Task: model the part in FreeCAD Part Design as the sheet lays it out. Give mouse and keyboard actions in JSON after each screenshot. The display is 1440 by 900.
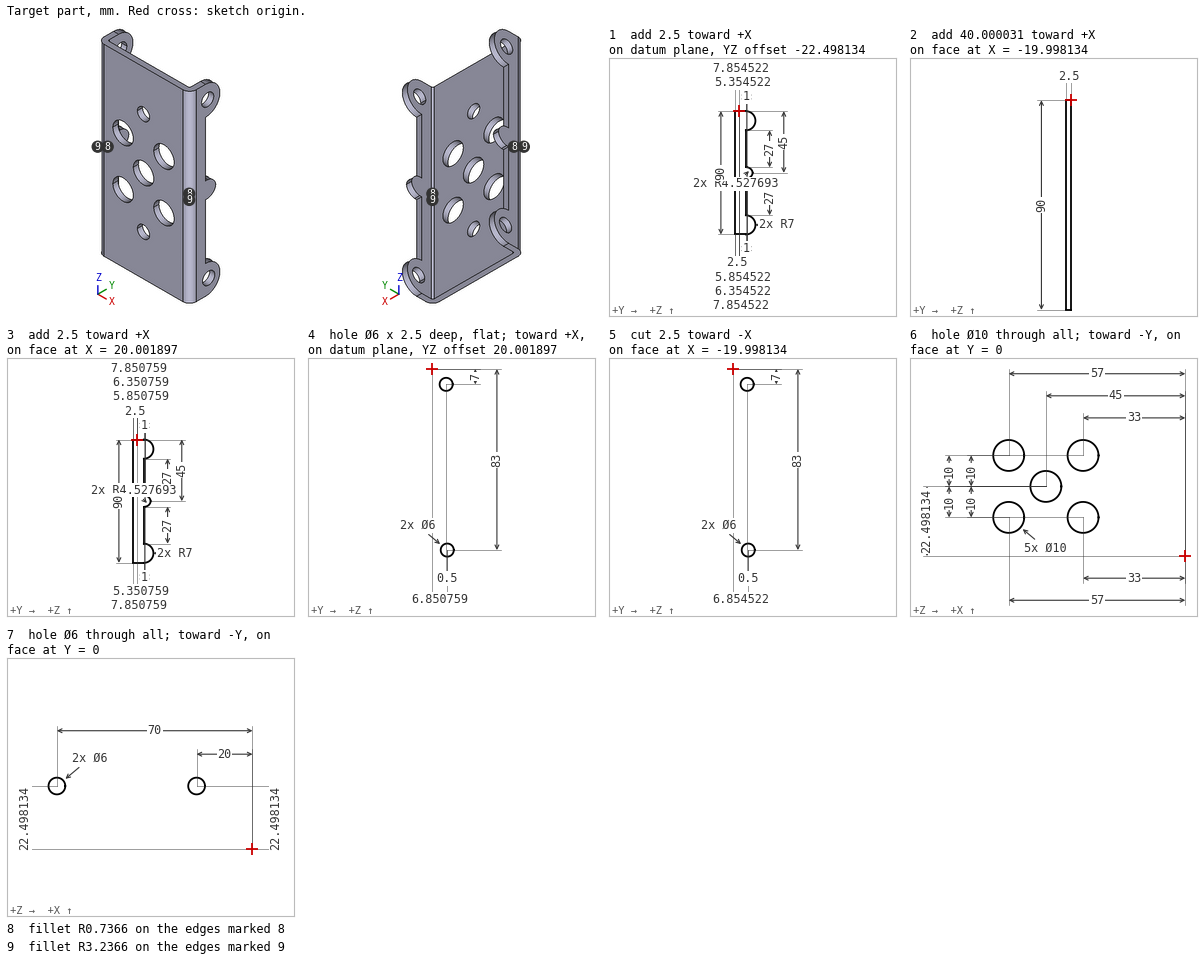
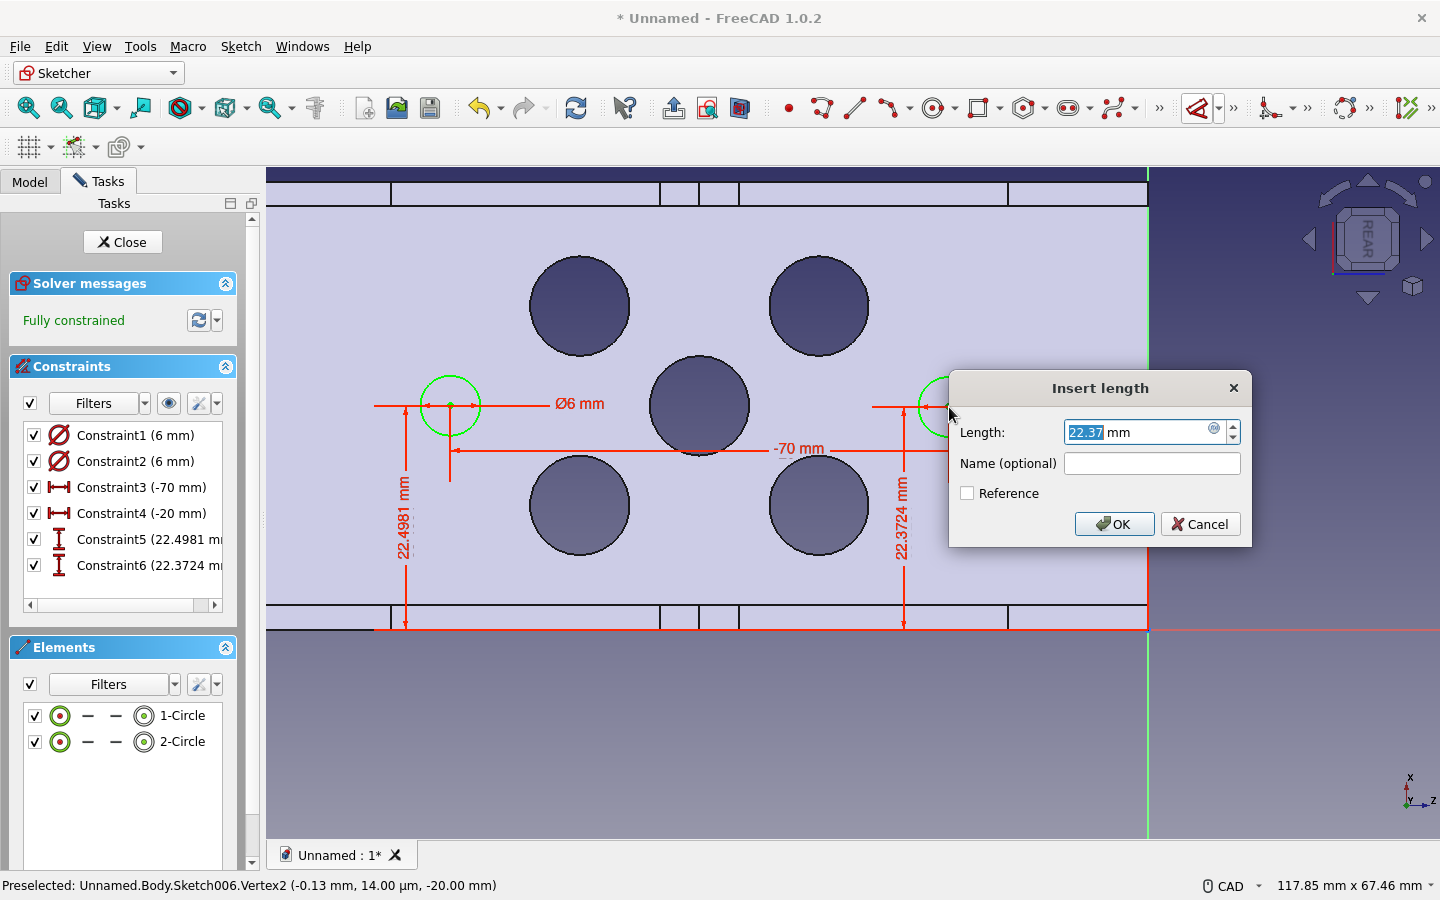
{"action": "type", "text": "22.498134"}
{"action": "key", "text": "Return"}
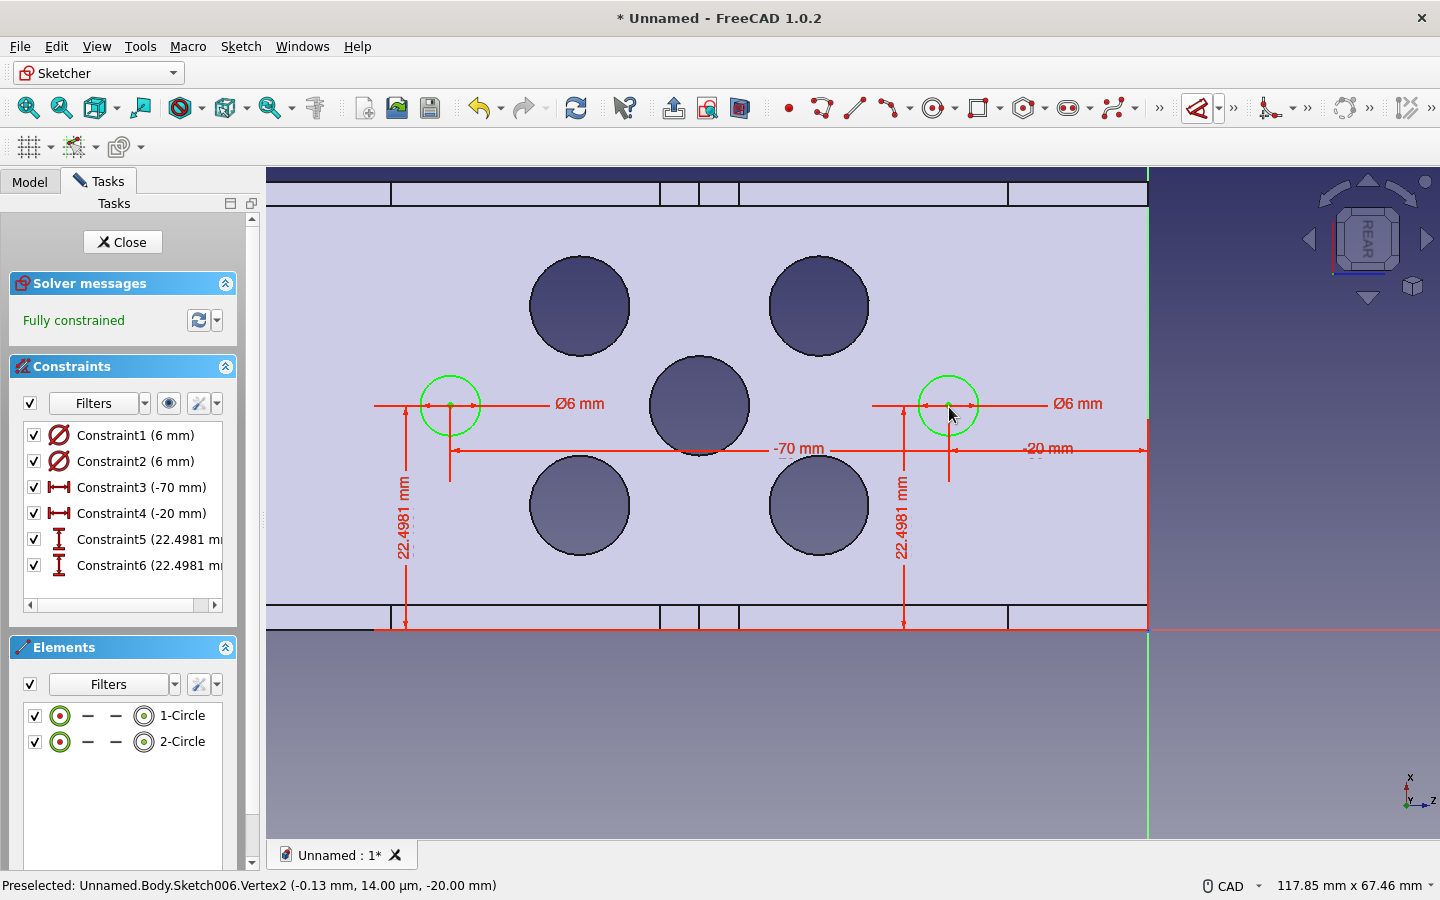
{"action": "left_click", "coordinate": [123, 242]}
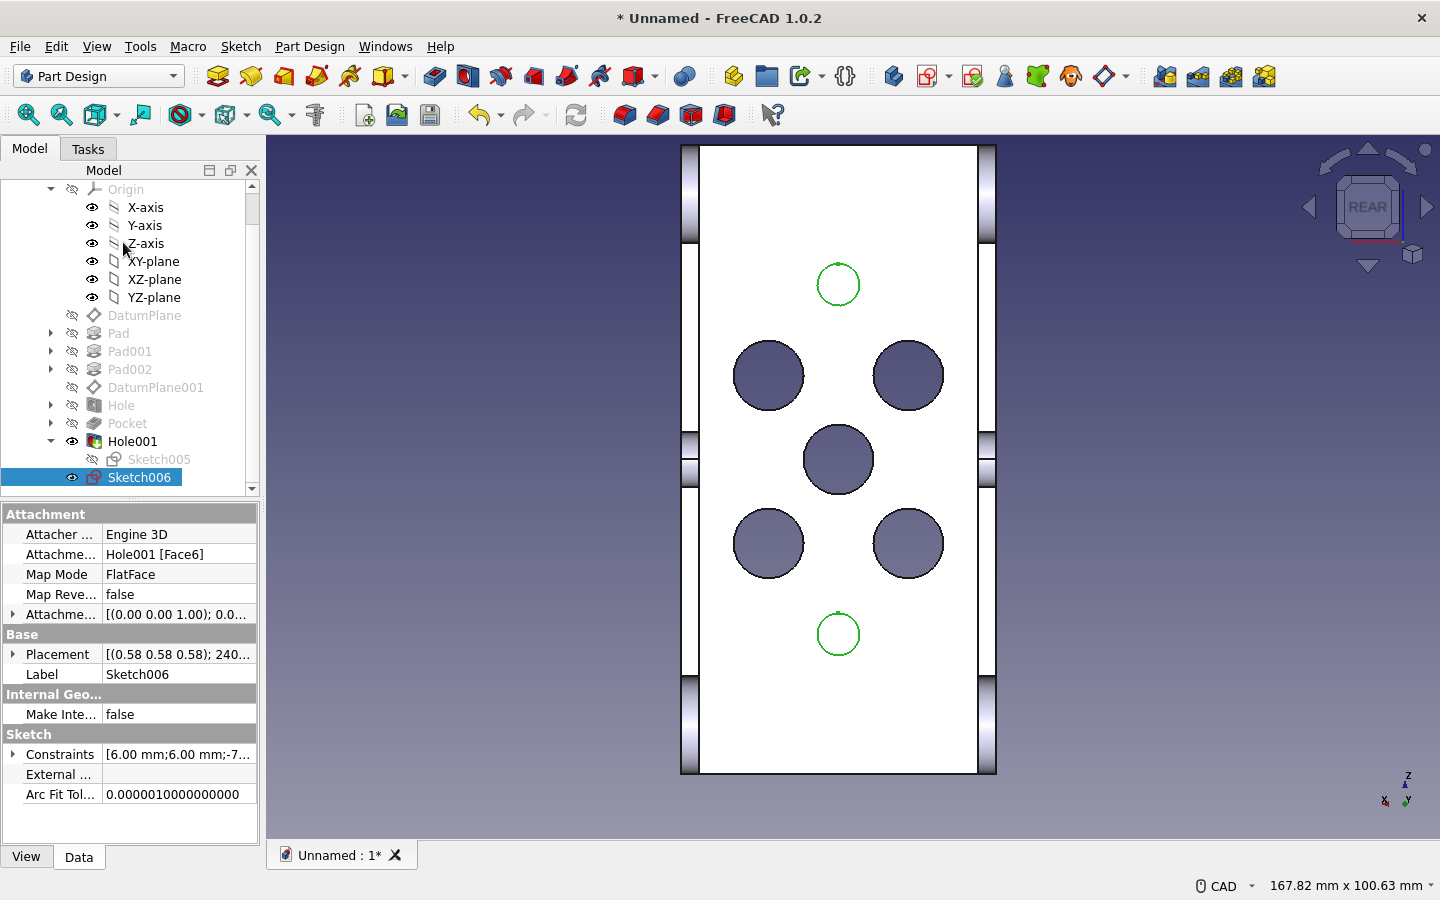
{"action": "left_click", "coordinate": [468, 76]}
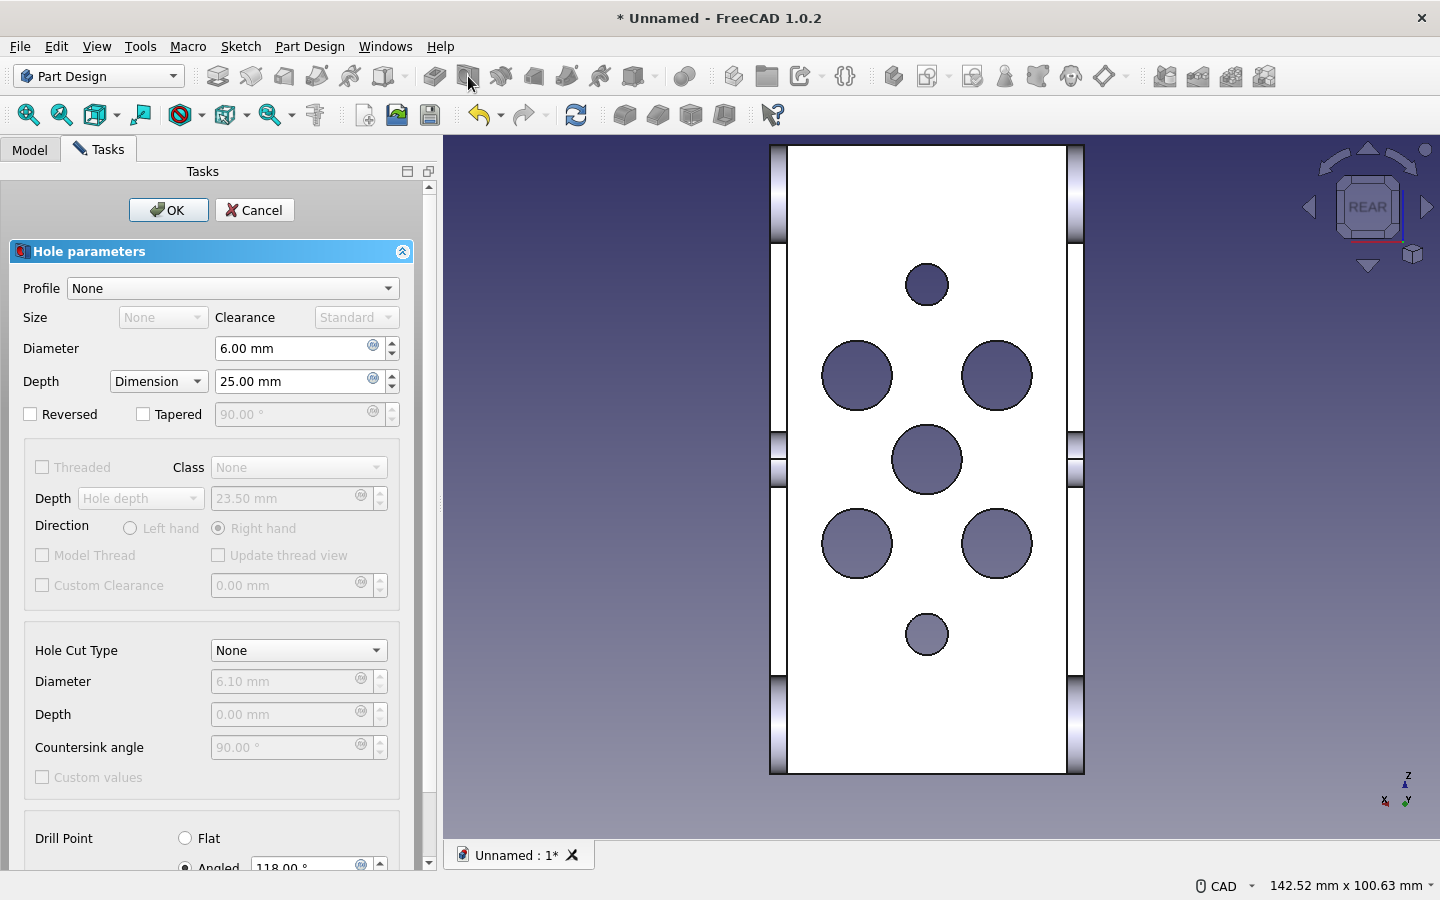
{"action": "triple_click", "coordinate": [300, 348]}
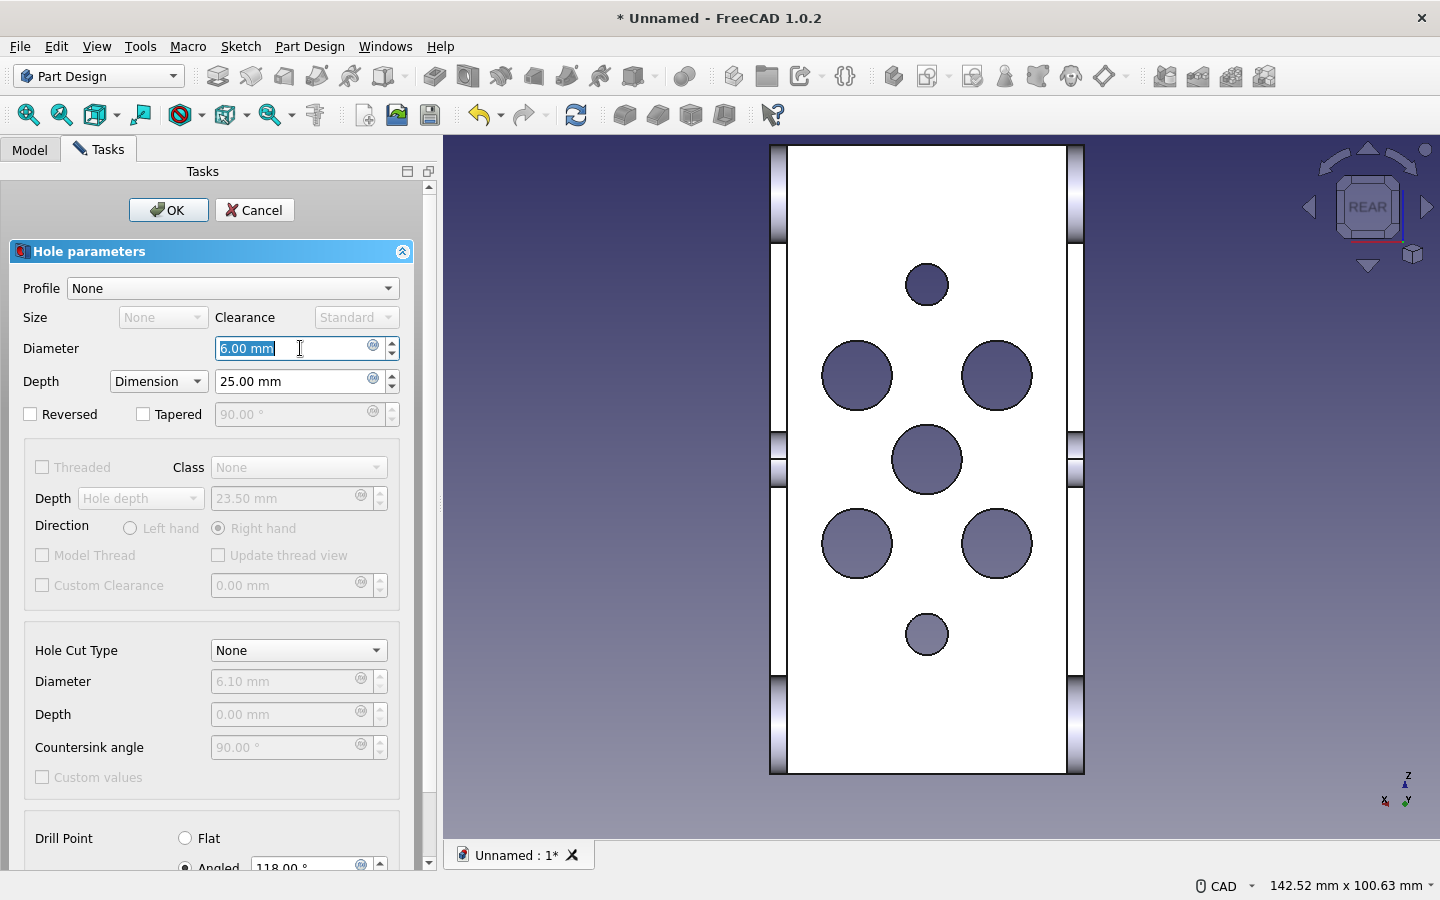
{"action": "type", "text": "6"}
{"action": "key", "text": "Tab"}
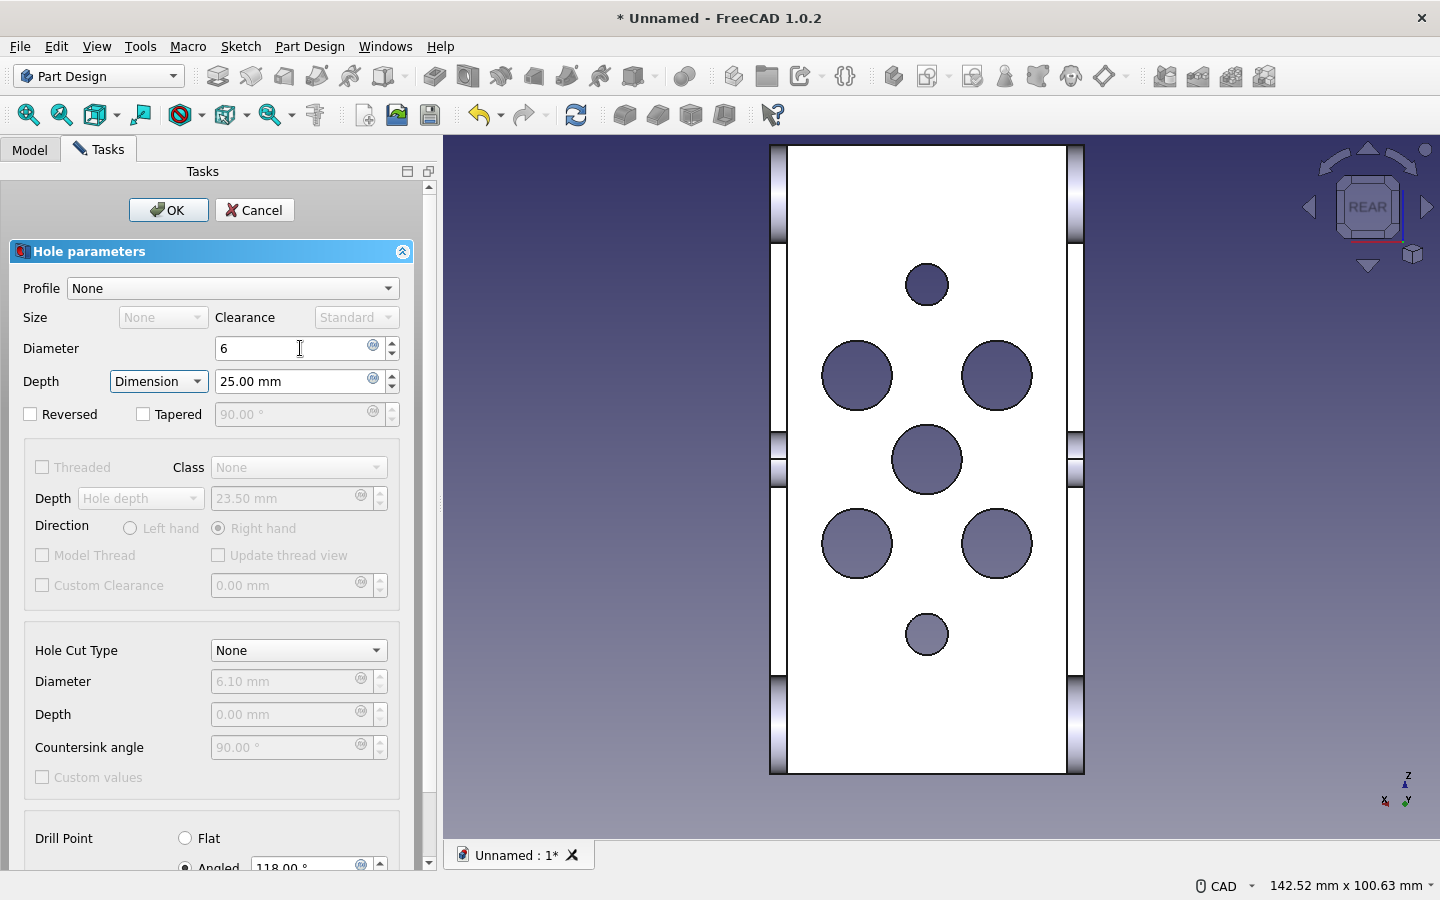
{"action": "left_click", "coordinate": [160, 382]}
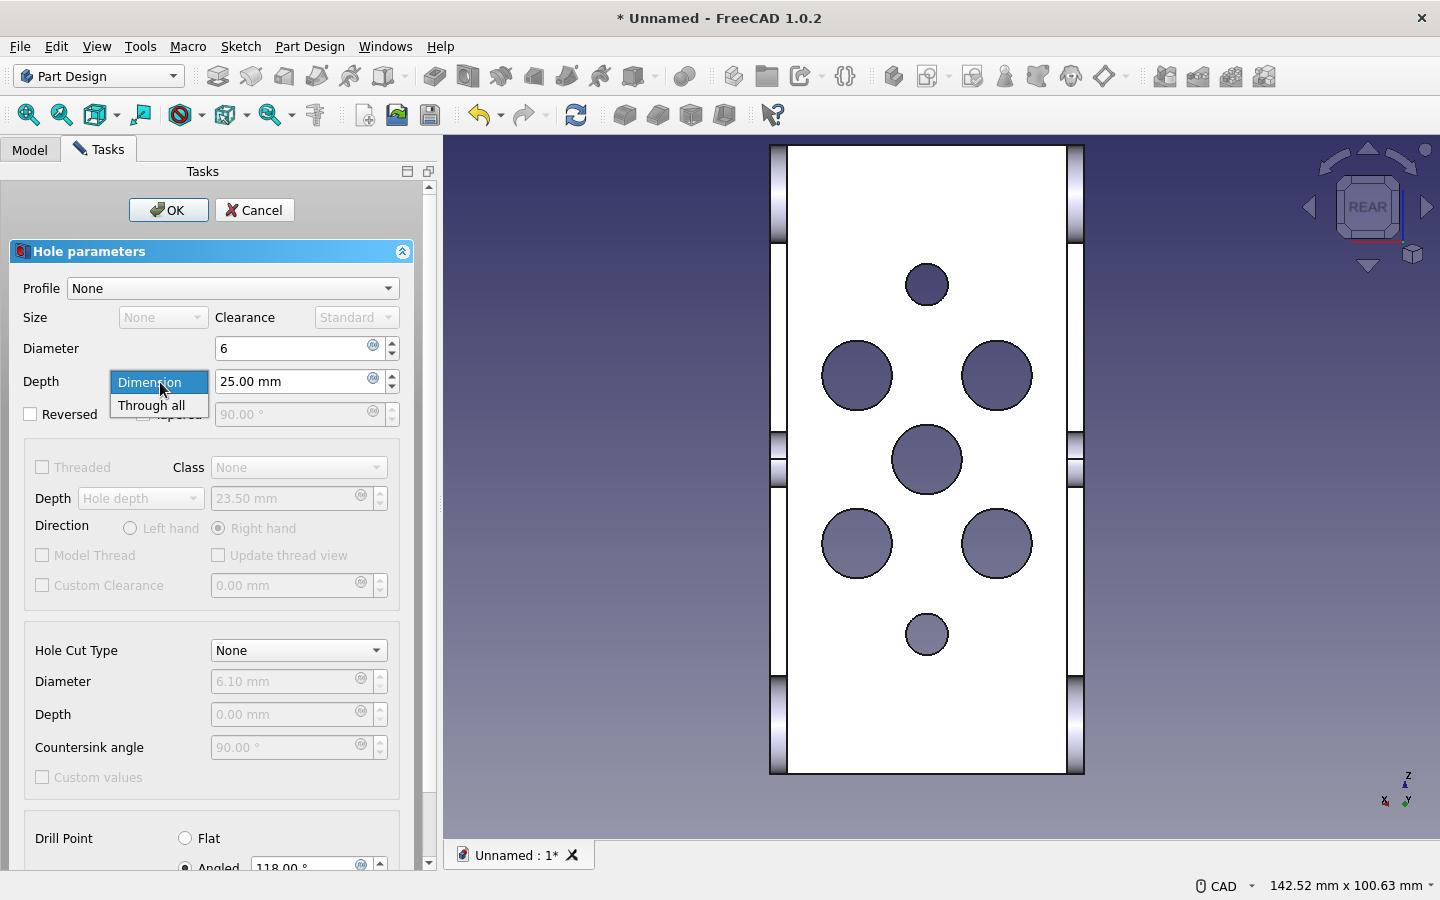
{"action": "left_click", "coordinate": [158, 406]}